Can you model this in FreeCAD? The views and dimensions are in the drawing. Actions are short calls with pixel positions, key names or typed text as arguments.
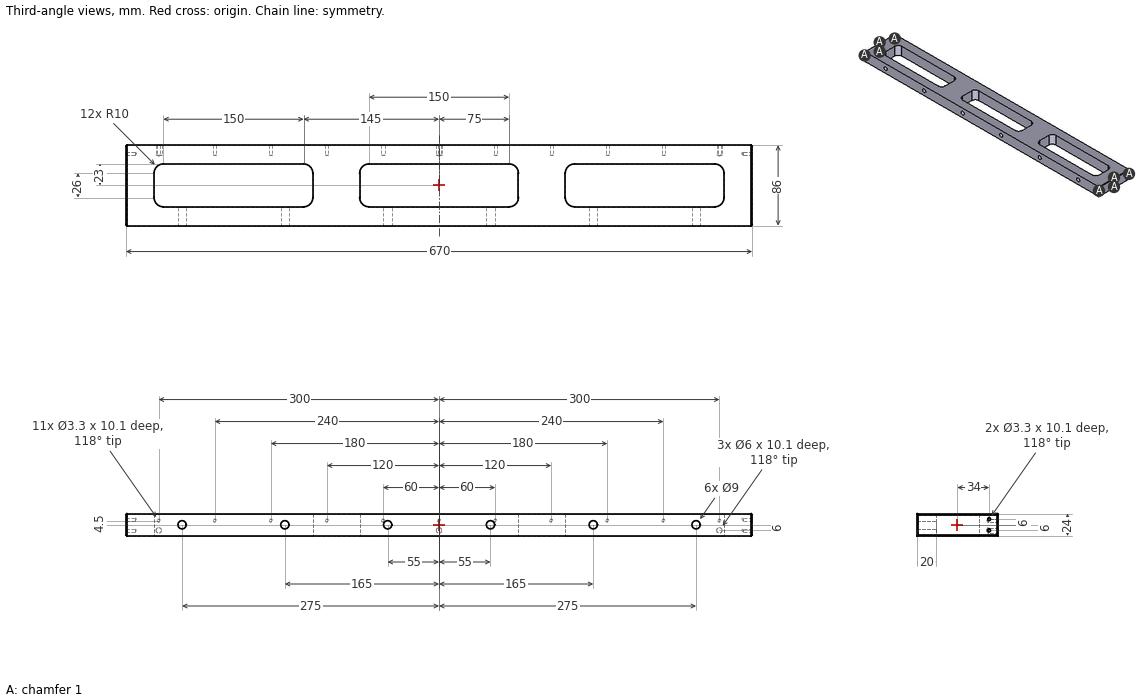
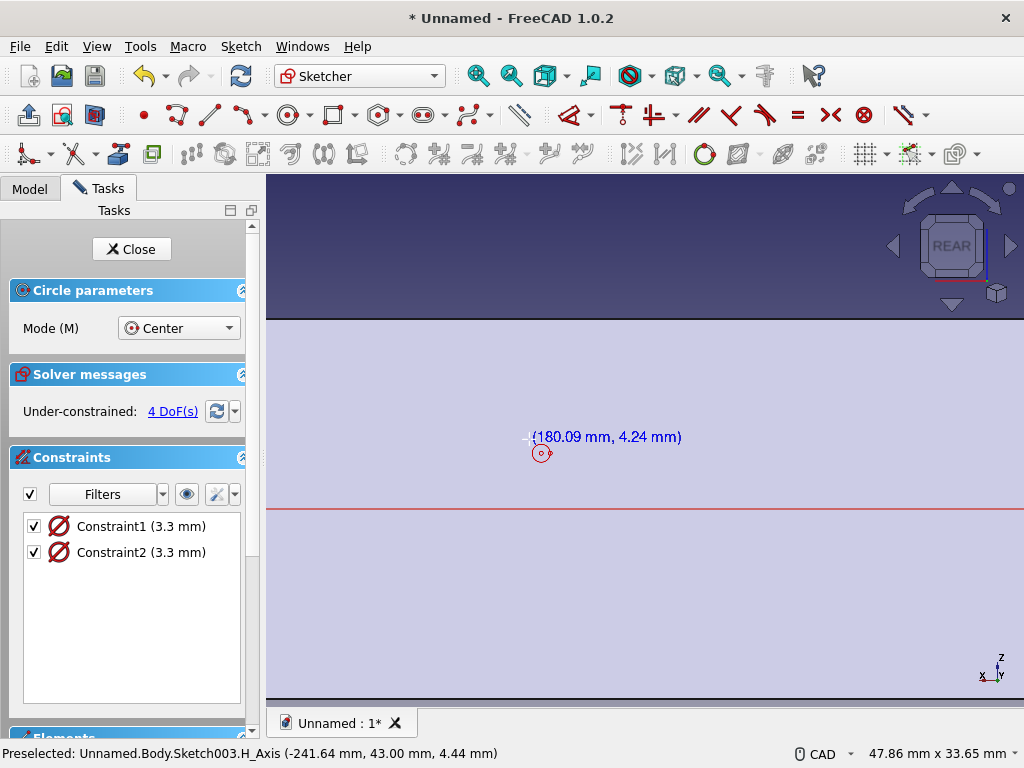
scroll(728, 439, down, 15)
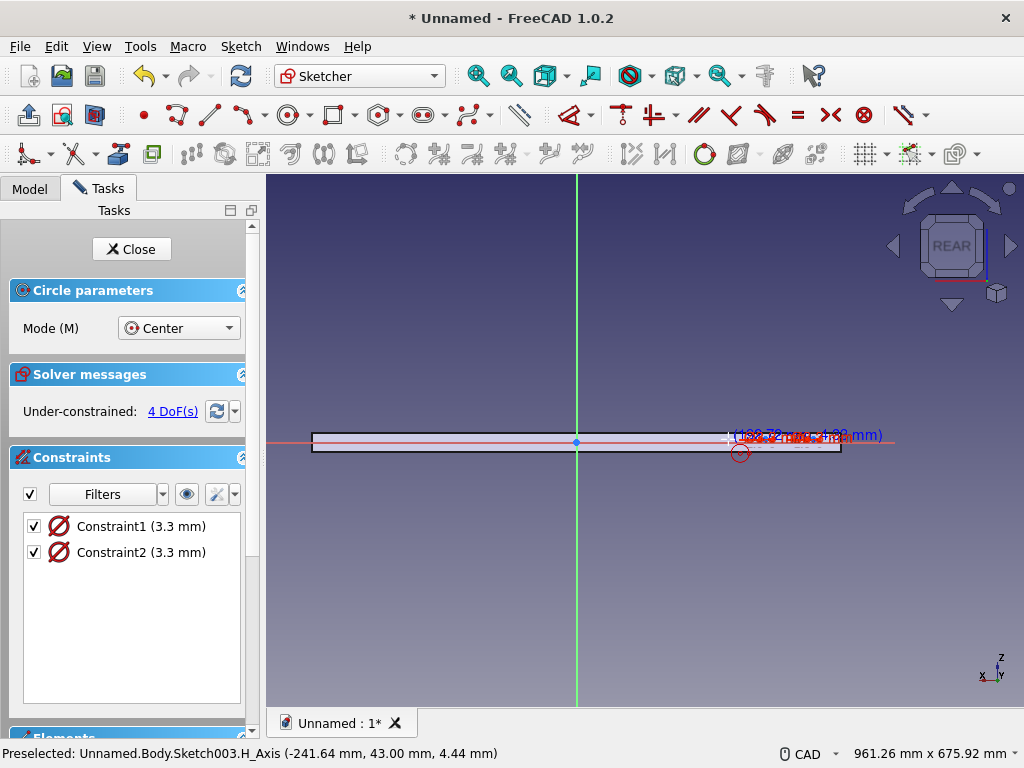
scroll(719, 439, up, 8)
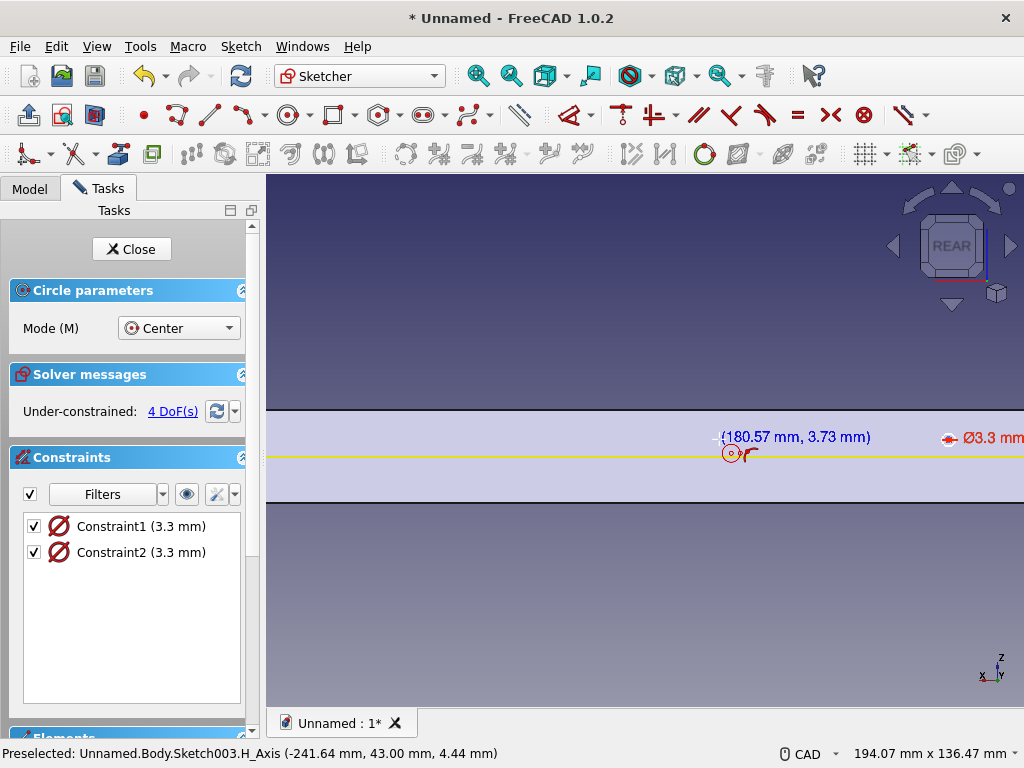
click(714, 439)
move(719, 434)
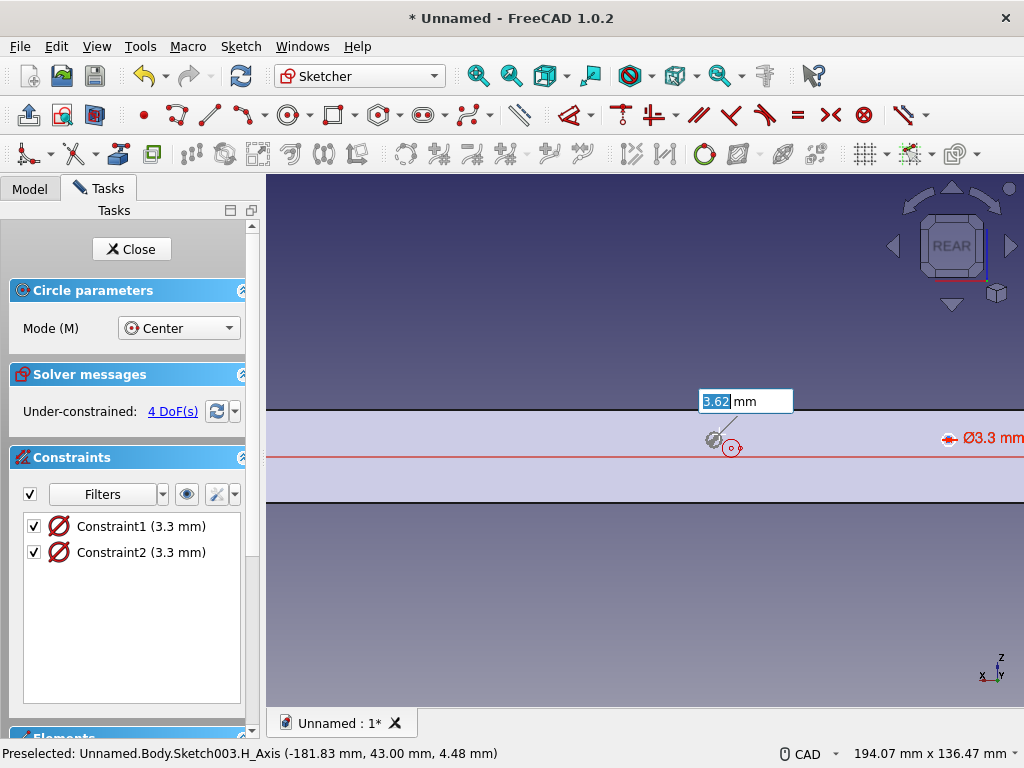
text(3.3)
key(Return)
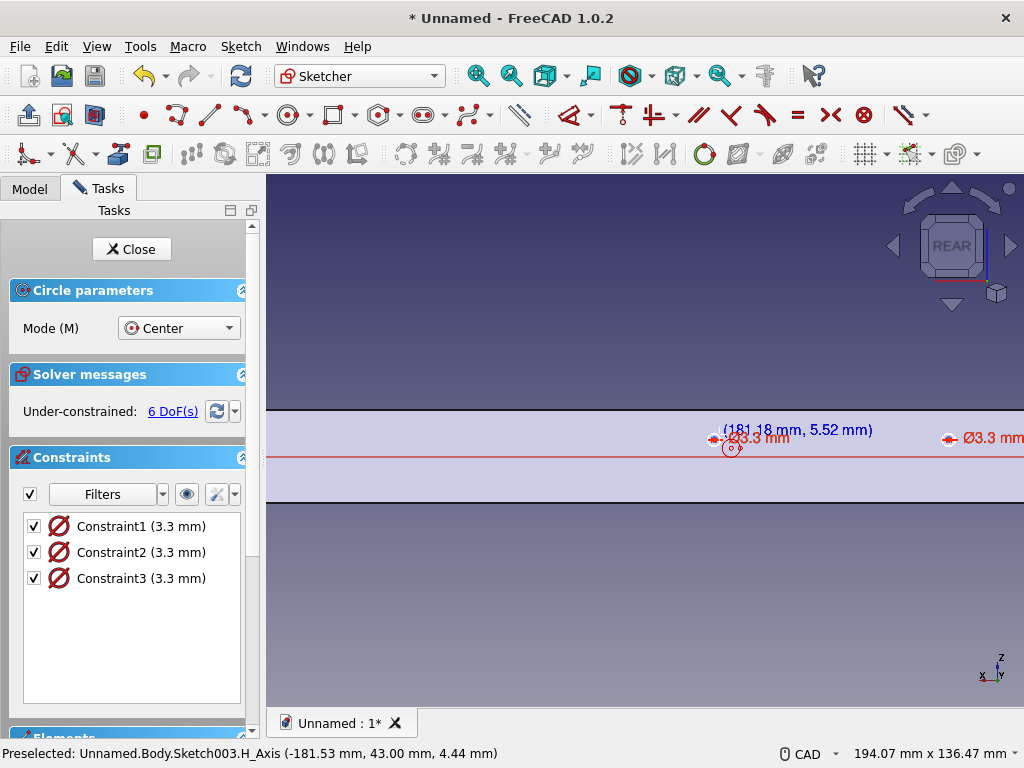
scroll(480, 439, up, 7)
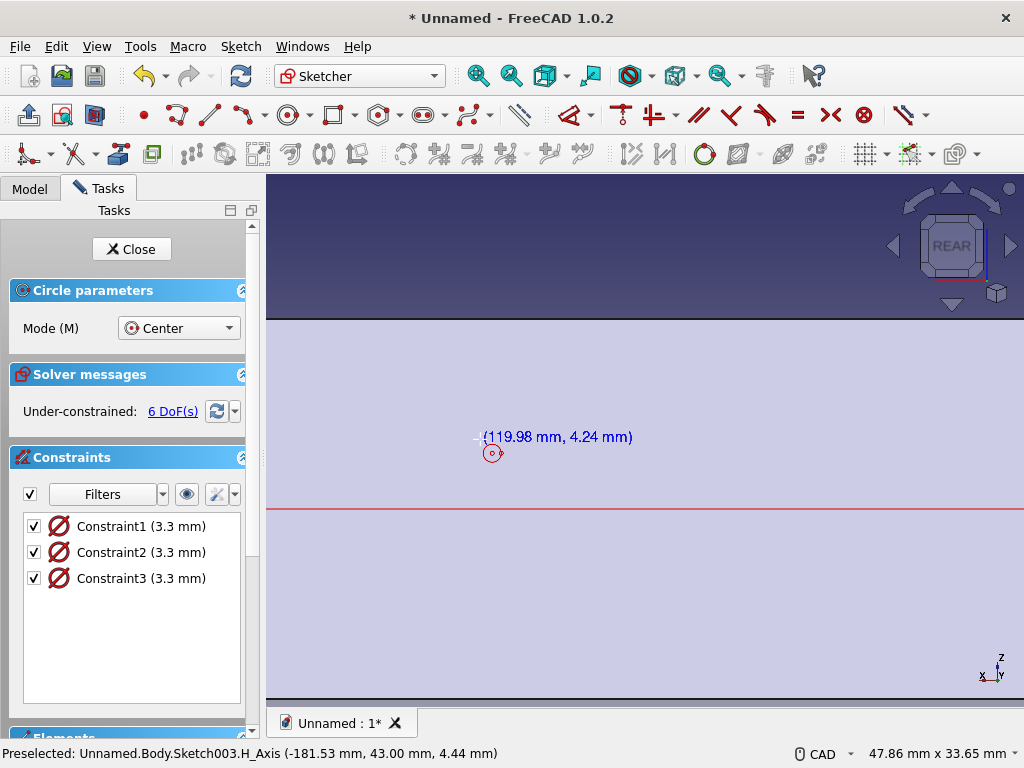
scroll(681, 439, down, 15)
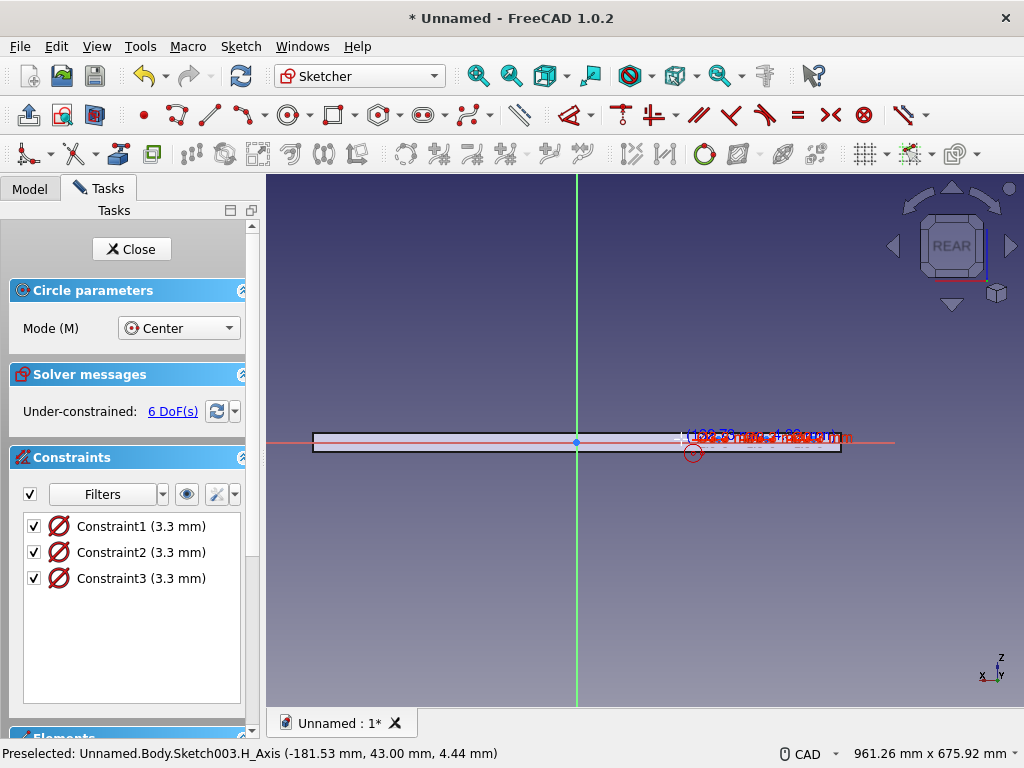
scroll(671, 439, up, 8)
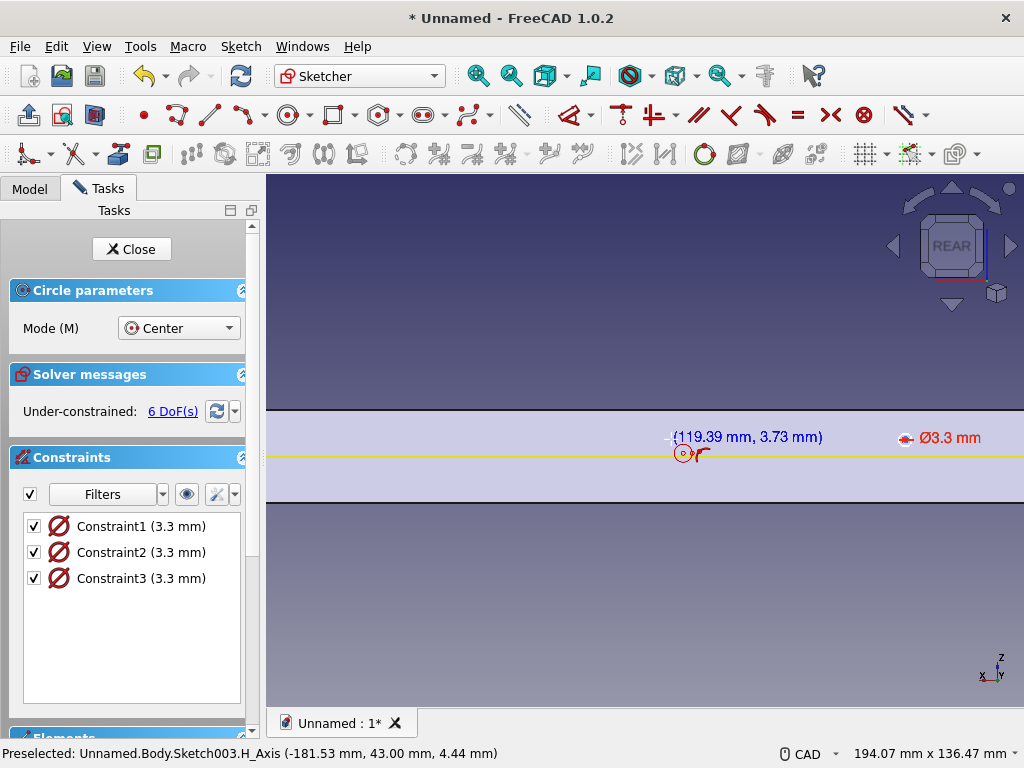
click(671, 439)
move(676, 434)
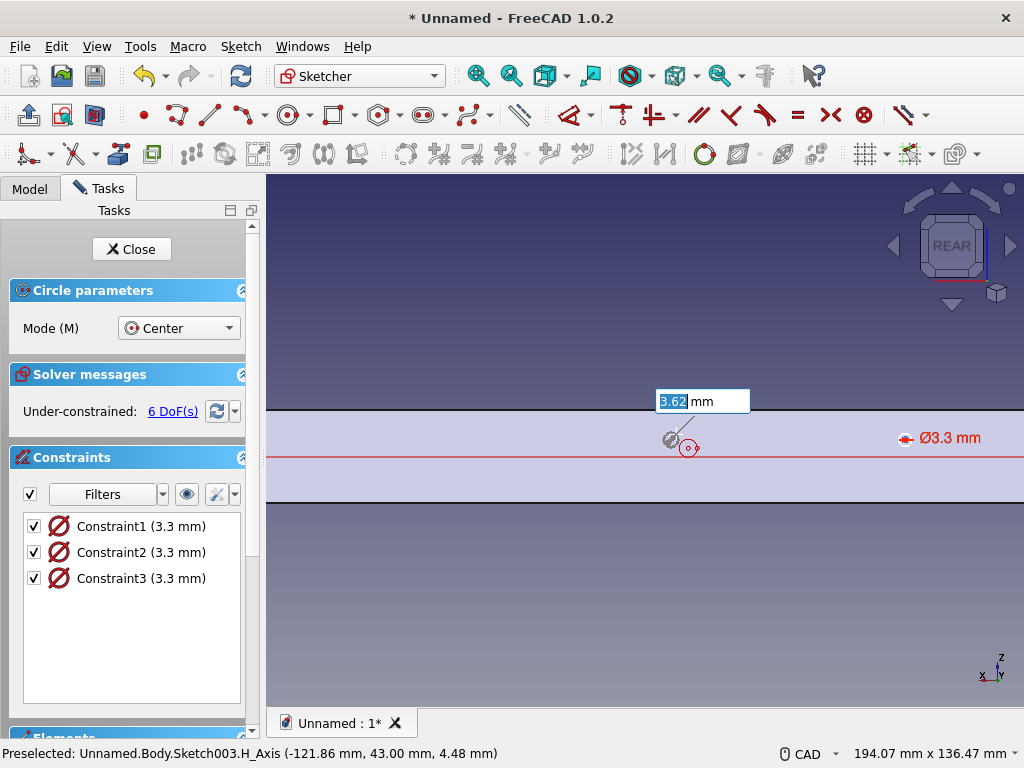
text(3.3)
key(Return)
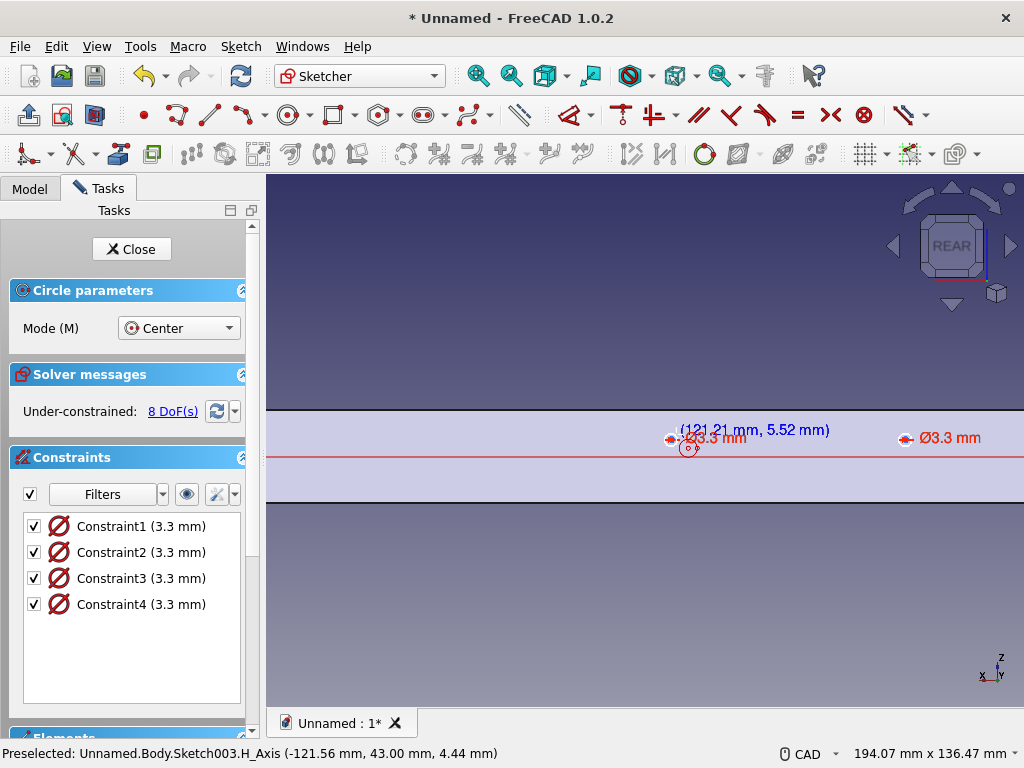
scroll(437, 439, up, 7)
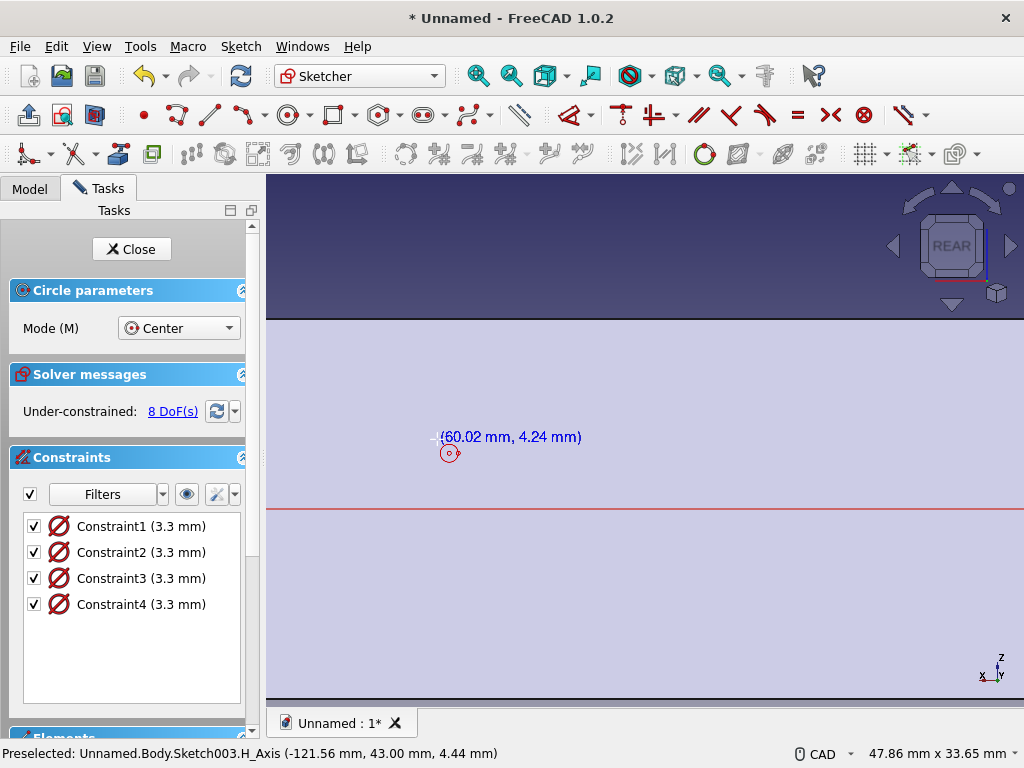
scroll(634, 439, down, 15)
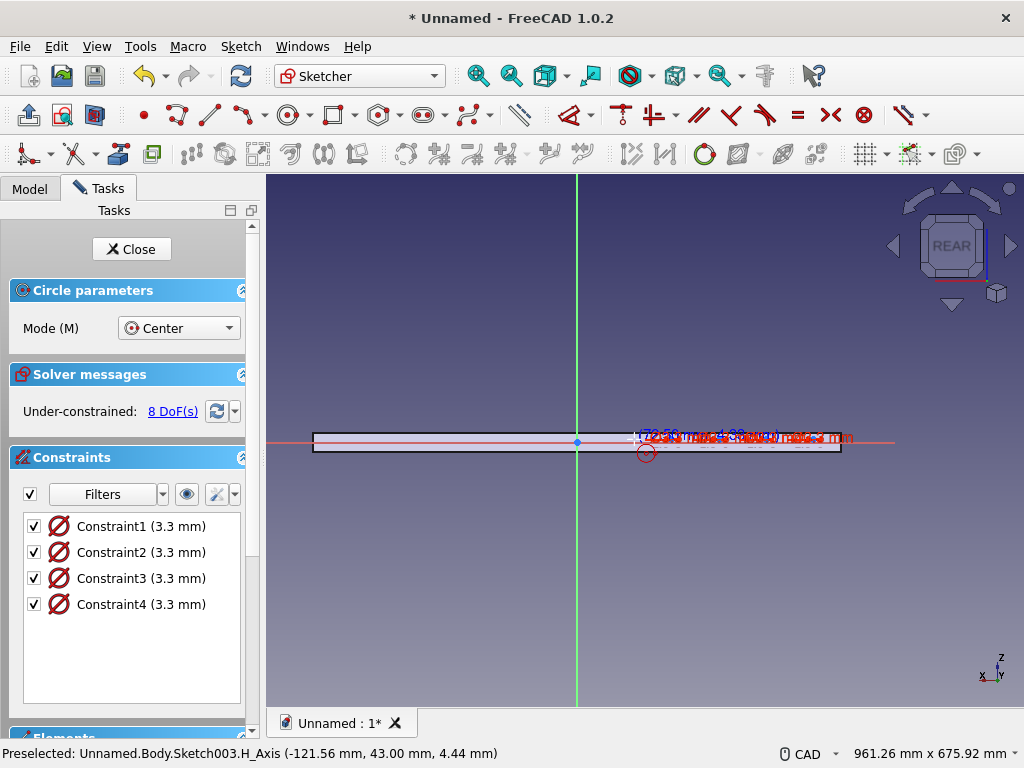
scroll(625, 439, up, 8)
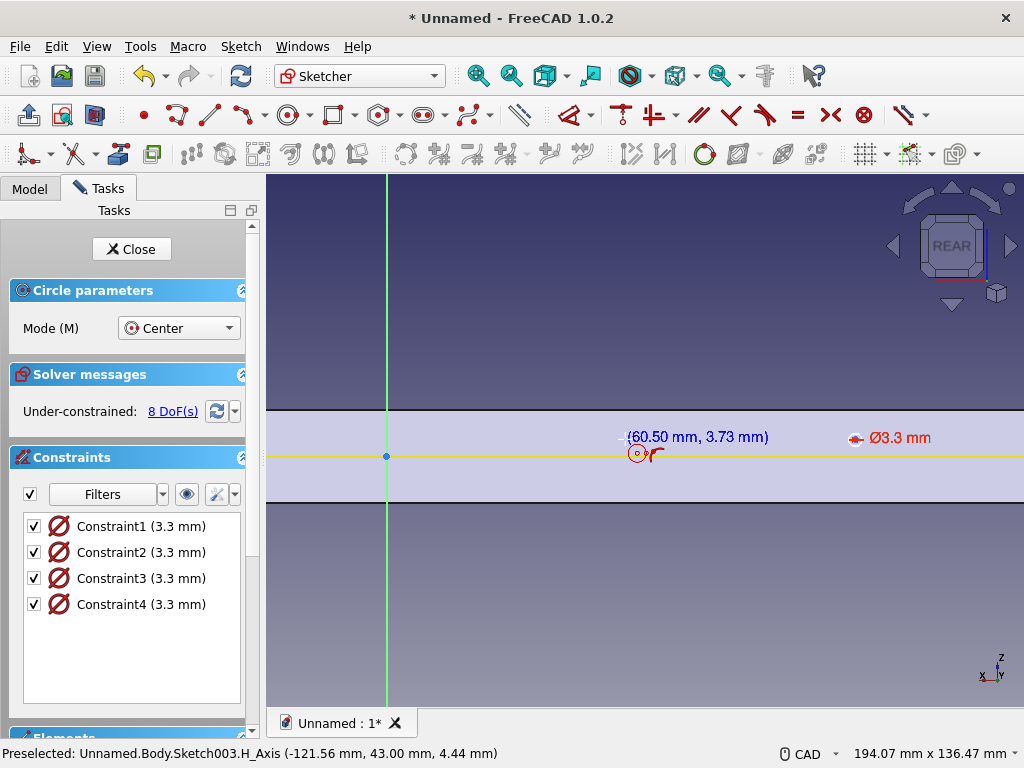
click(621, 439)
move(626, 434)